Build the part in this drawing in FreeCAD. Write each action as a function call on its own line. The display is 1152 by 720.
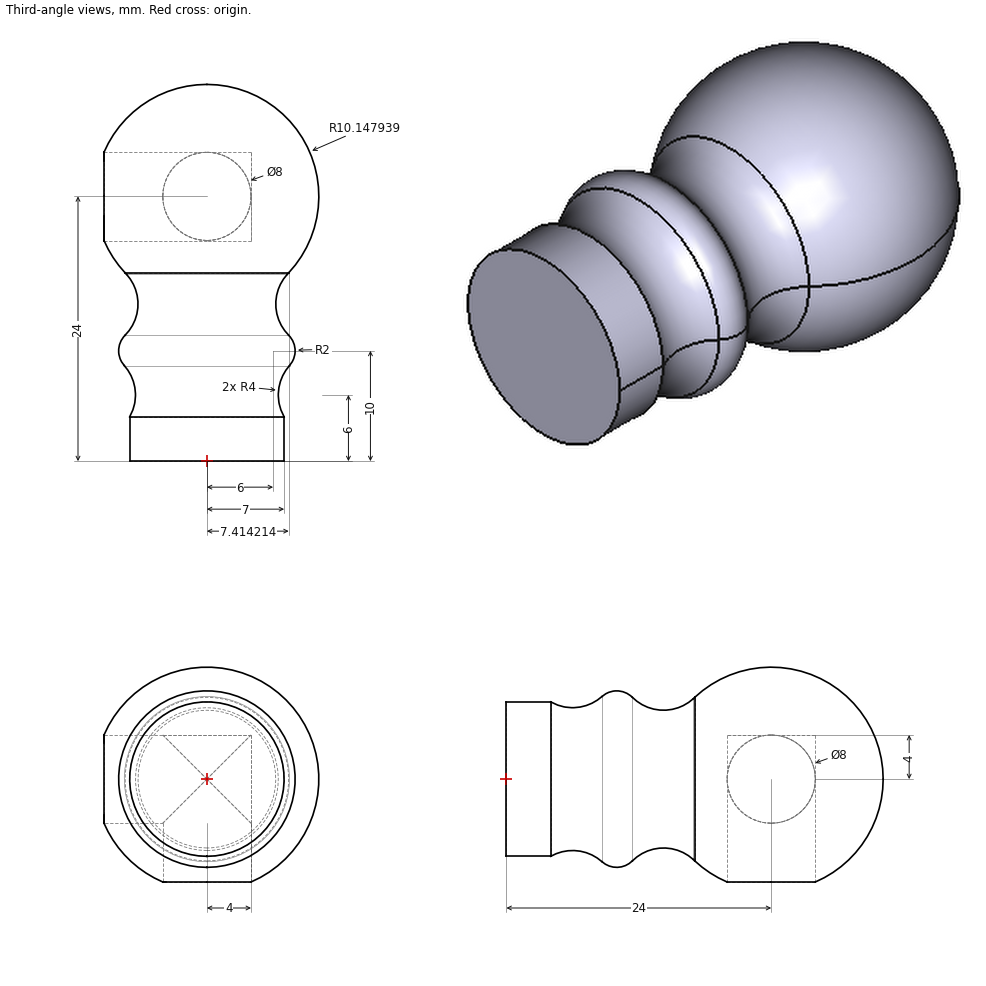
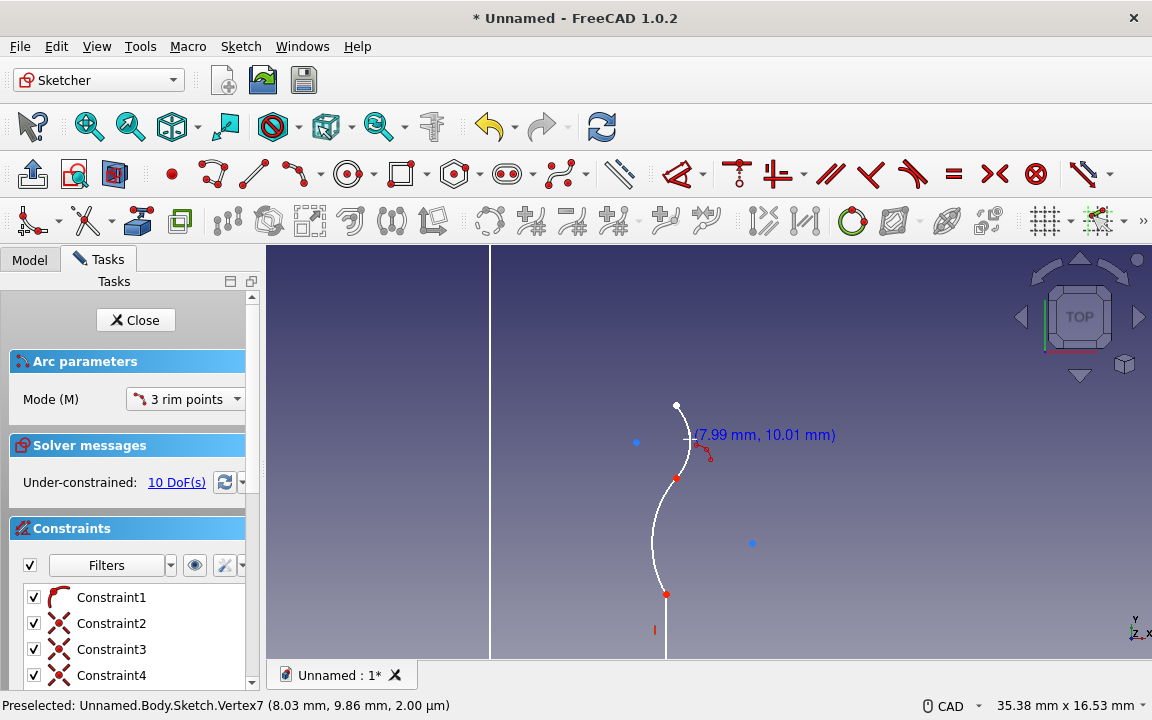
click(676, 406)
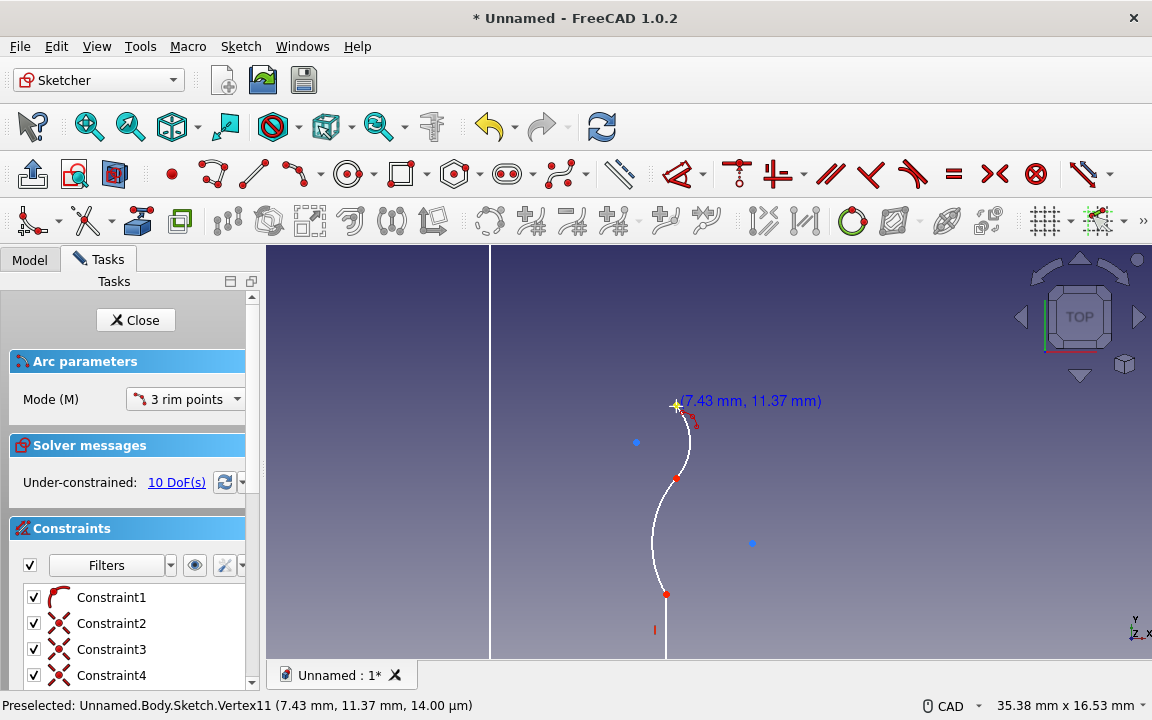
scroll(655, 533, down, 6)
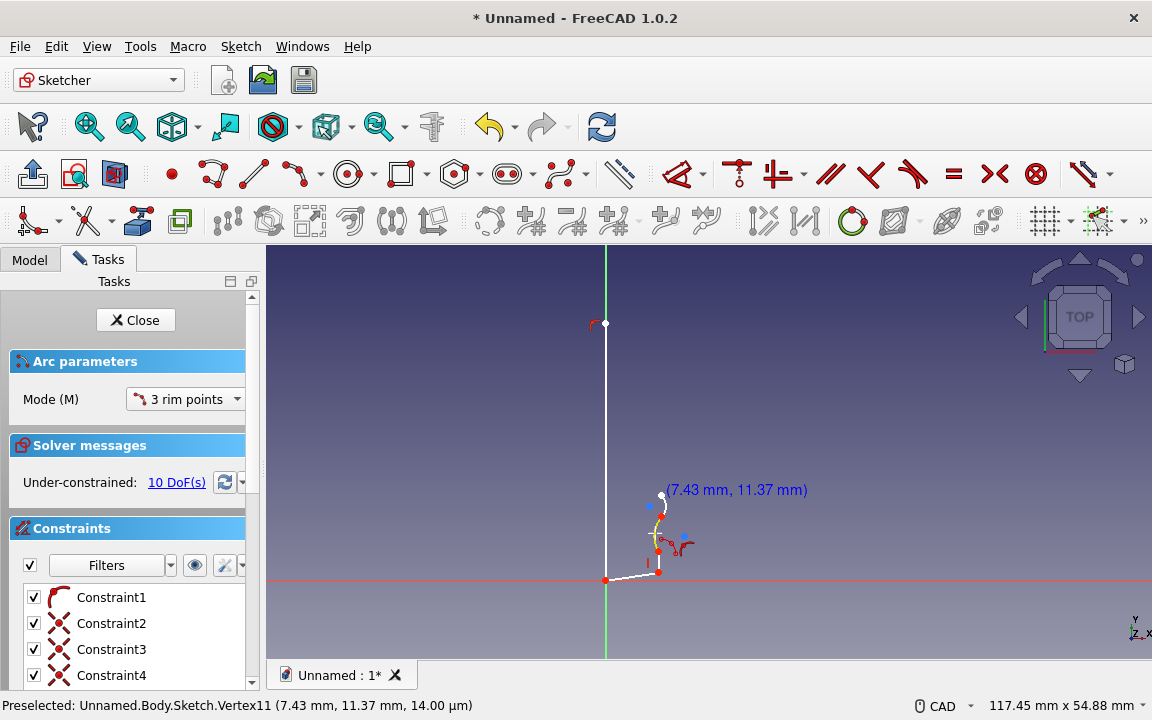
click(662, 452)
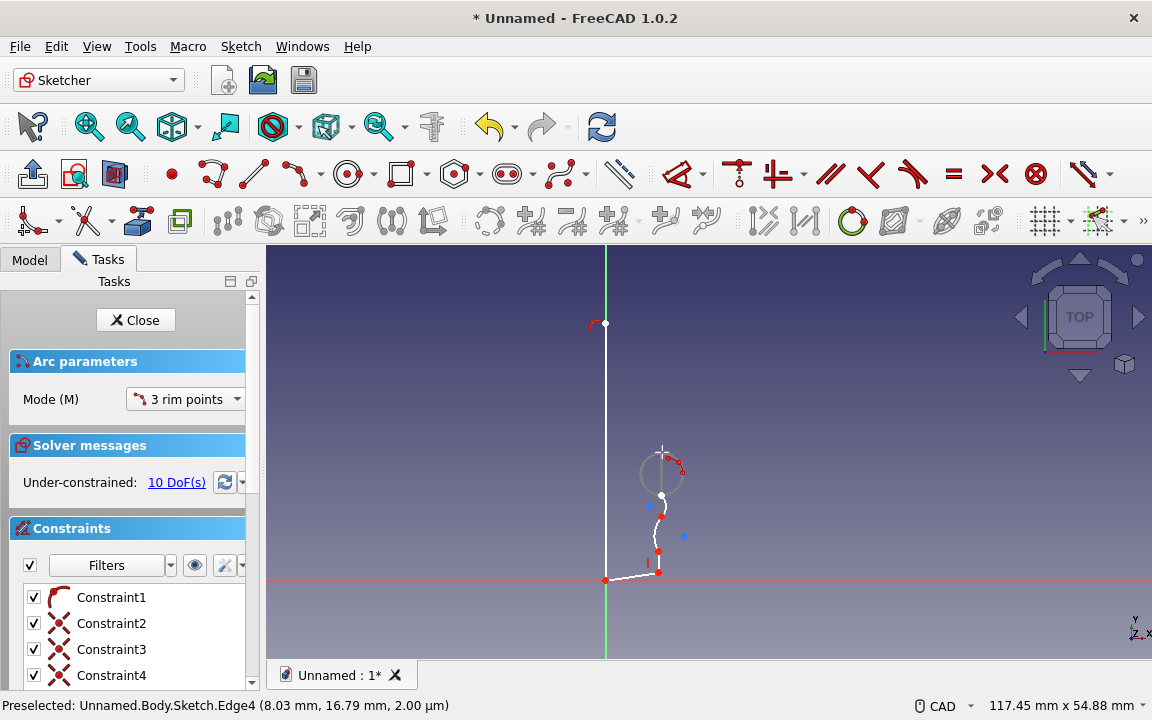
scroll(653, 474, up, 3)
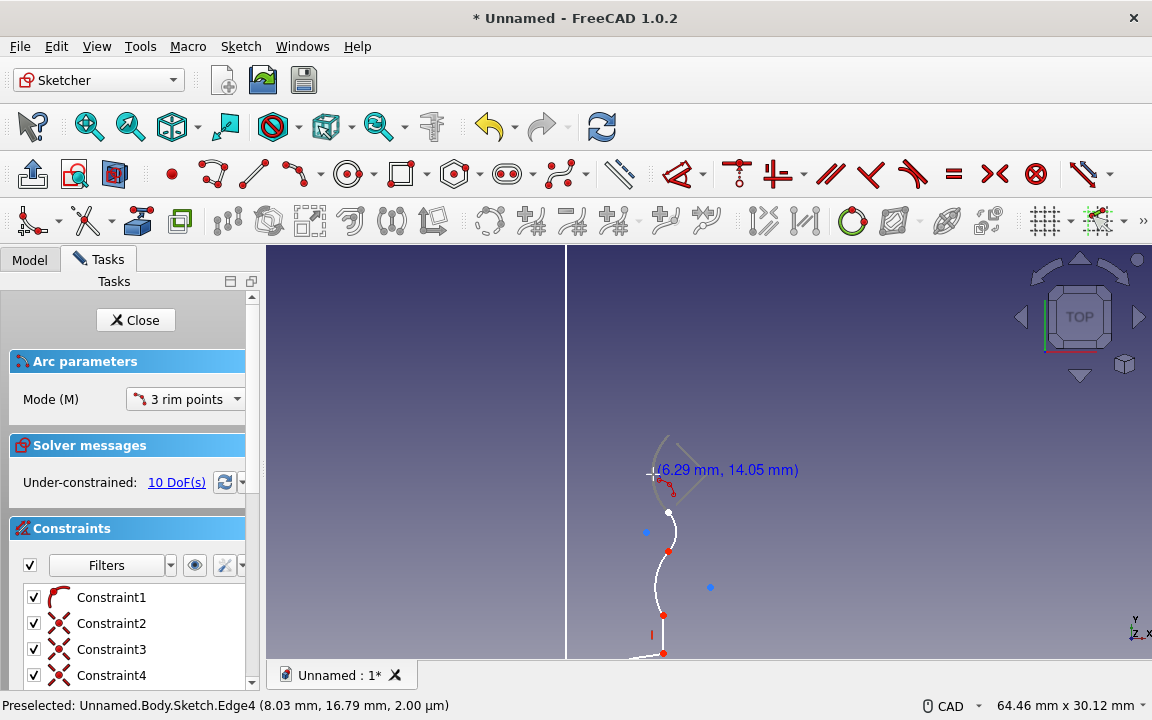
click(652, 473)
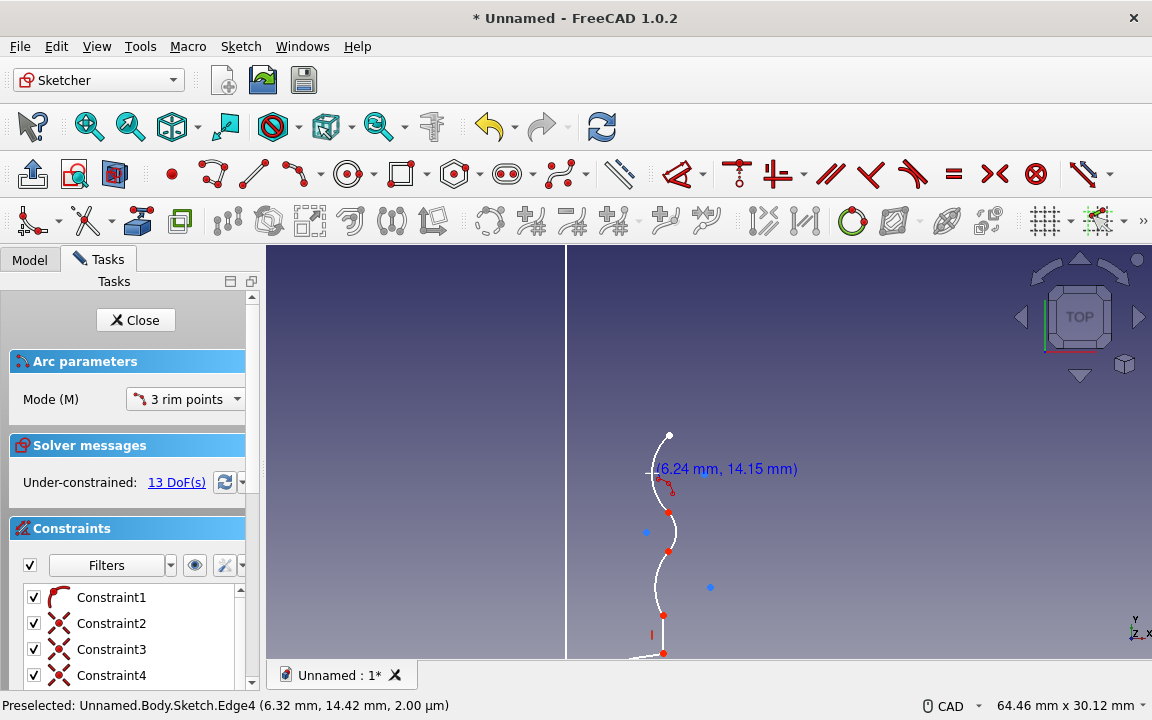
click(669, 435)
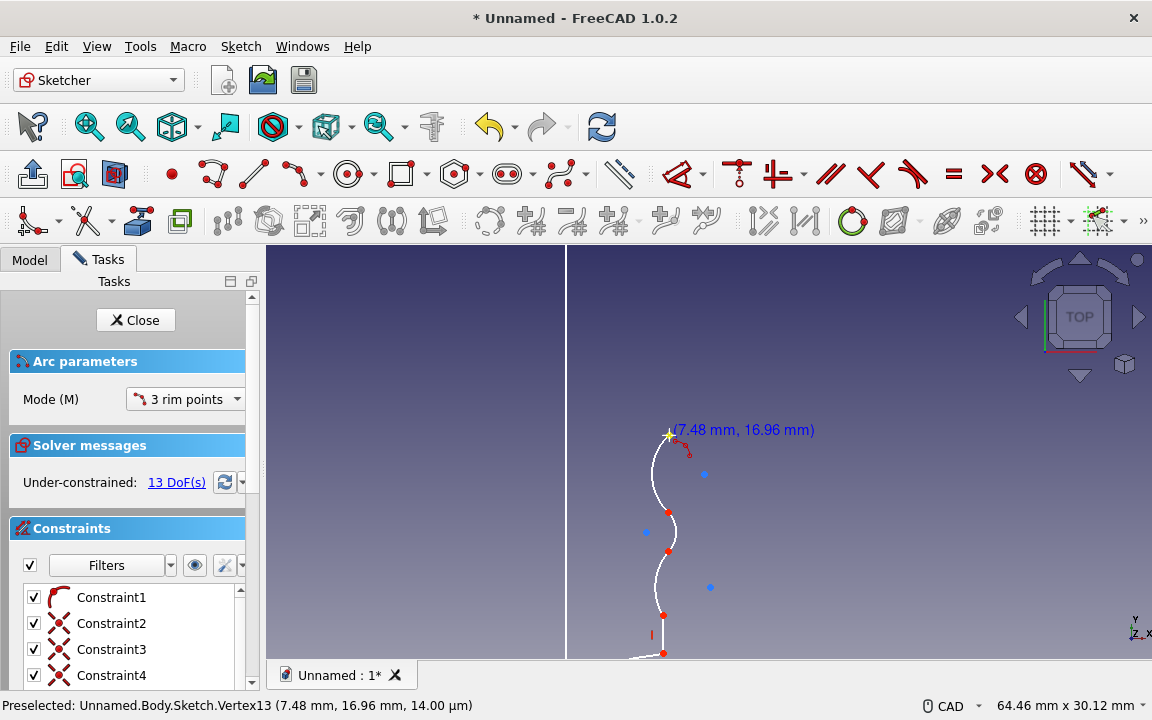
scroll(653, 474, down, 3)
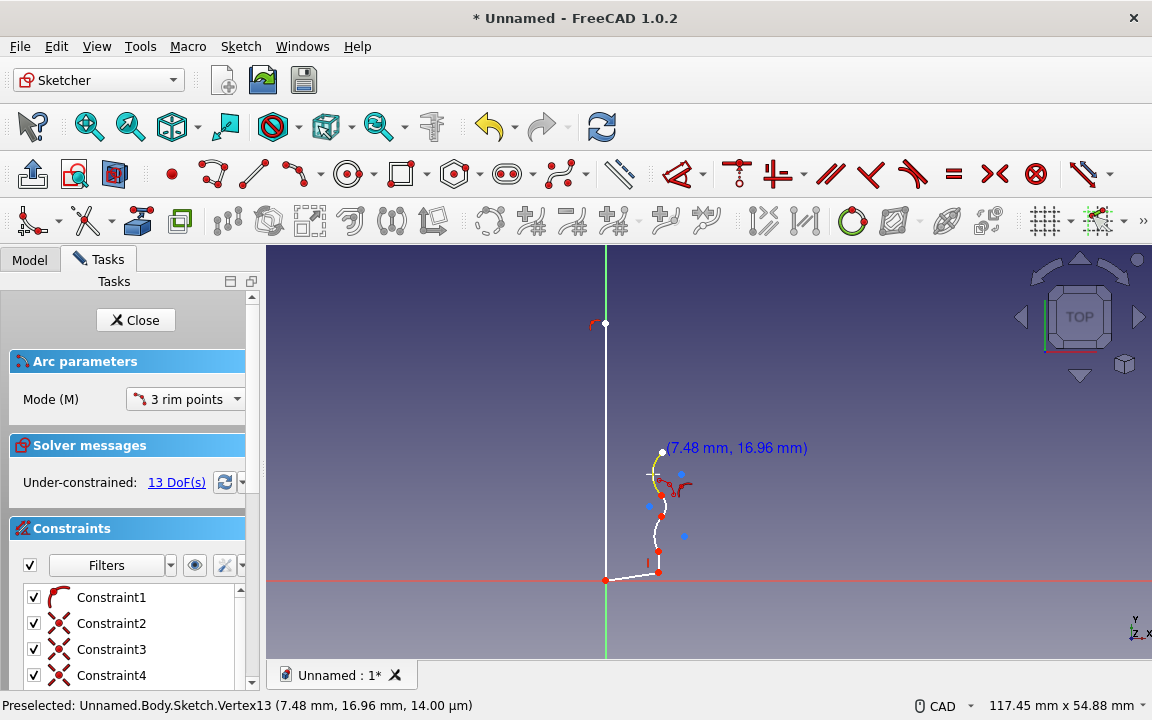
click(606, 324)
click(676, 369)
key(Escape)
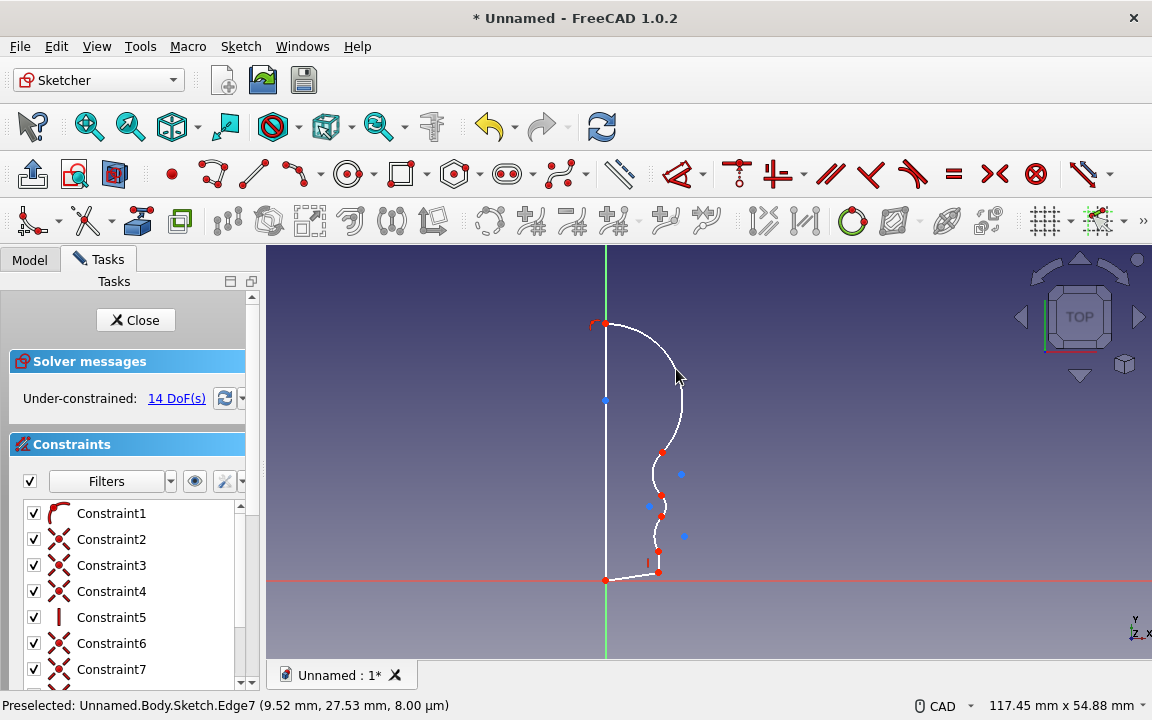
scroll(656, 527, up, 2)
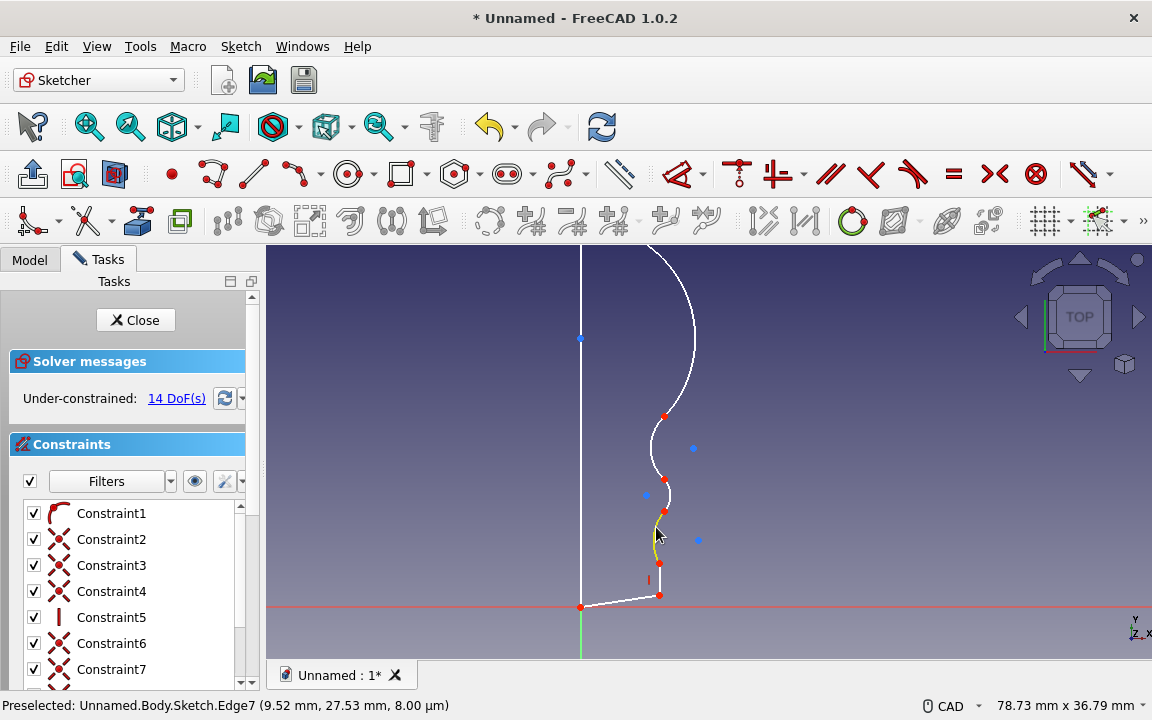
click(656, 526)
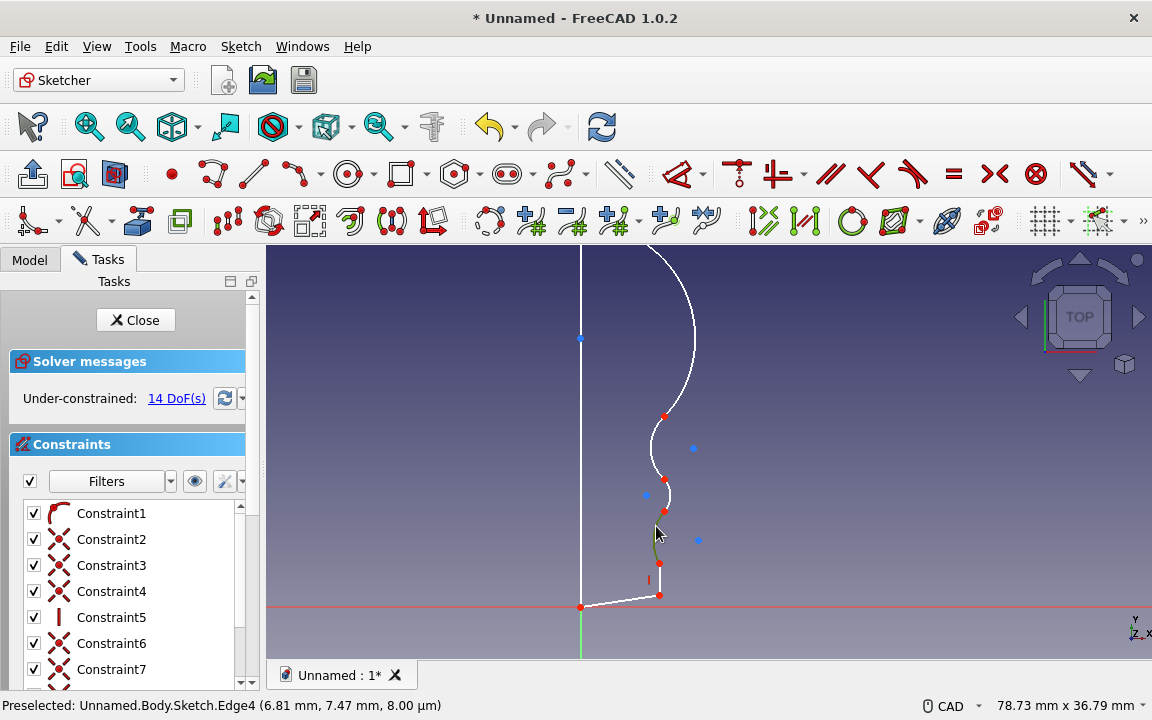
scroll(669, 503, up, 2)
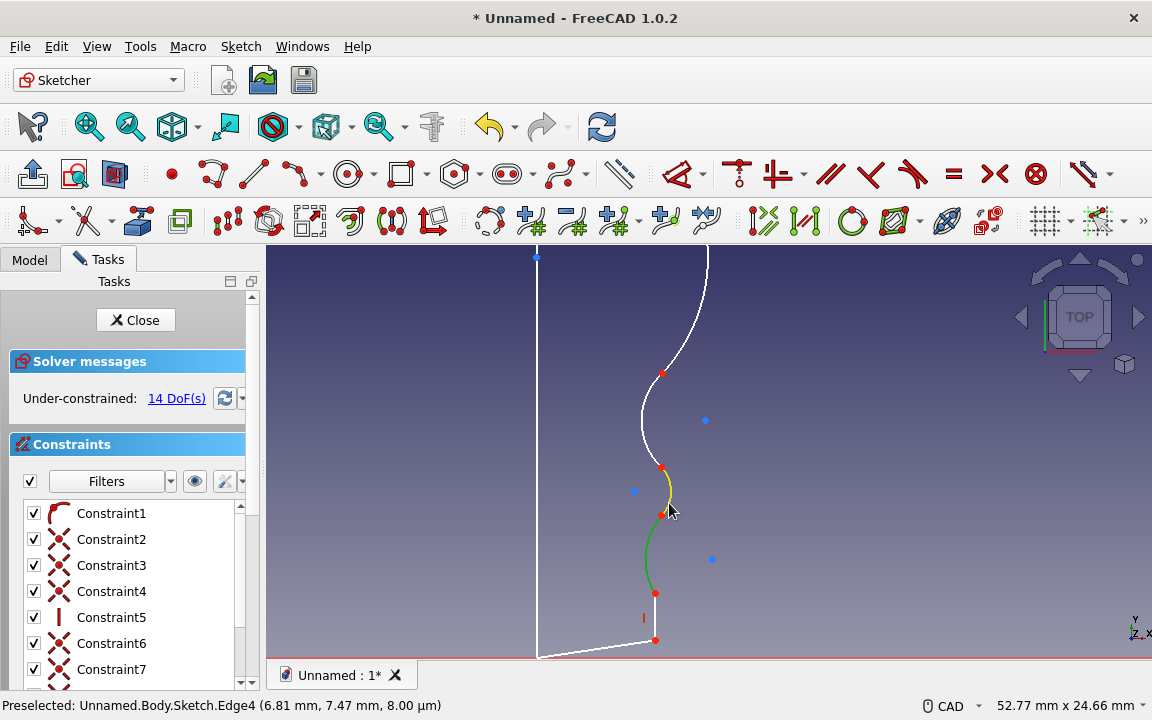
click(669, 502)